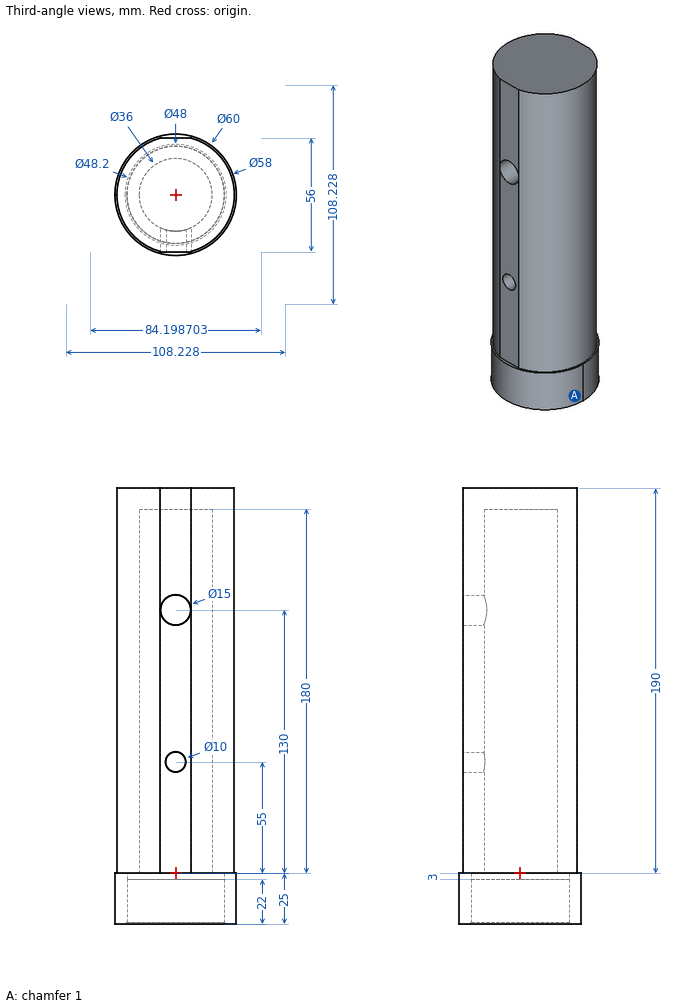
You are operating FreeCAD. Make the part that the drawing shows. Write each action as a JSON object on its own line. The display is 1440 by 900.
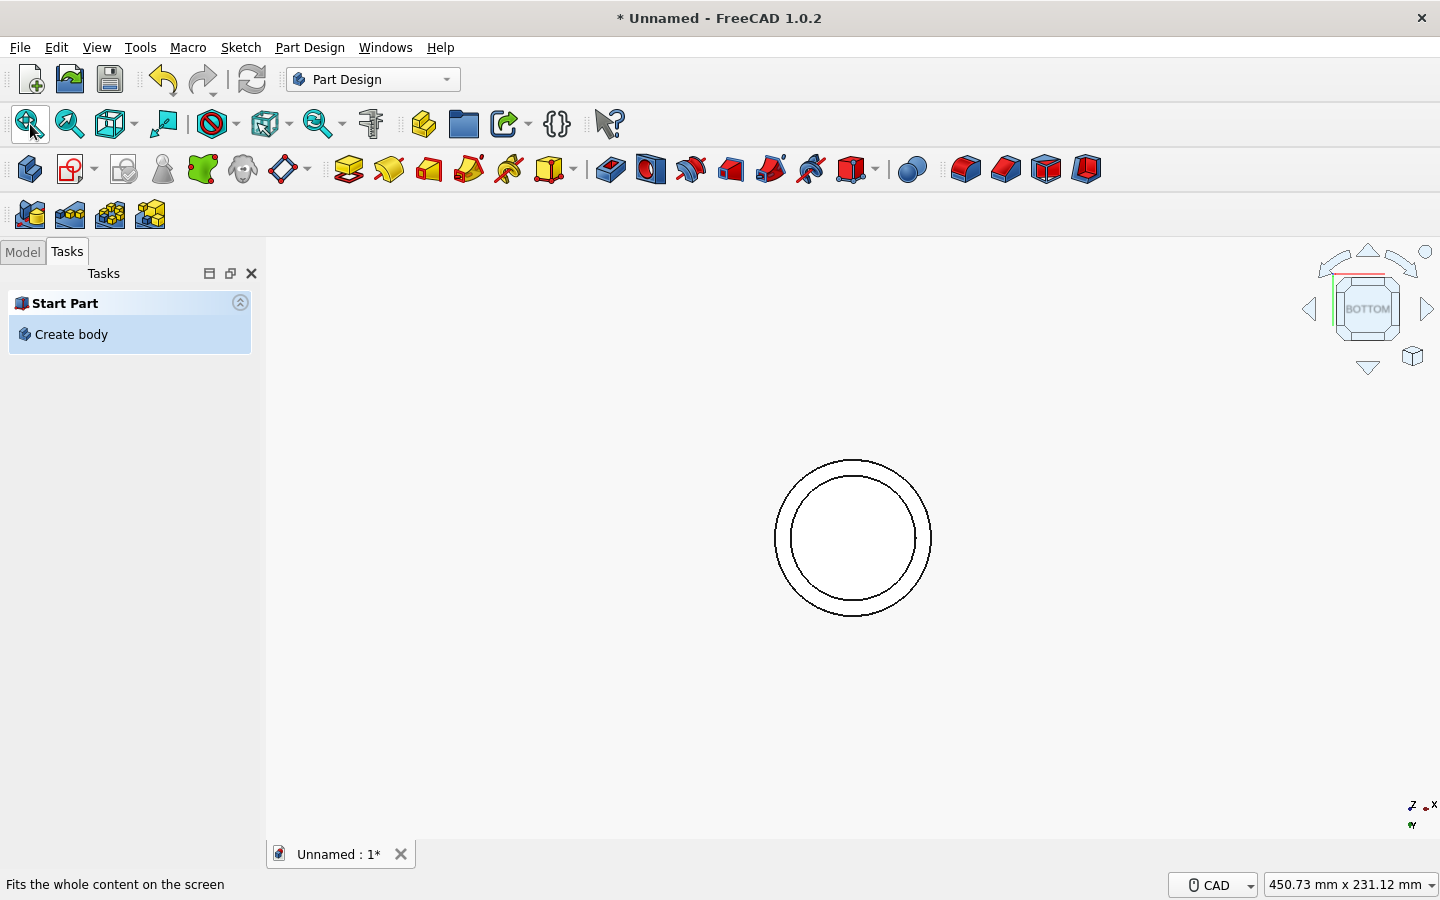
{"action": "left_click", "coordinate": [853, 537]}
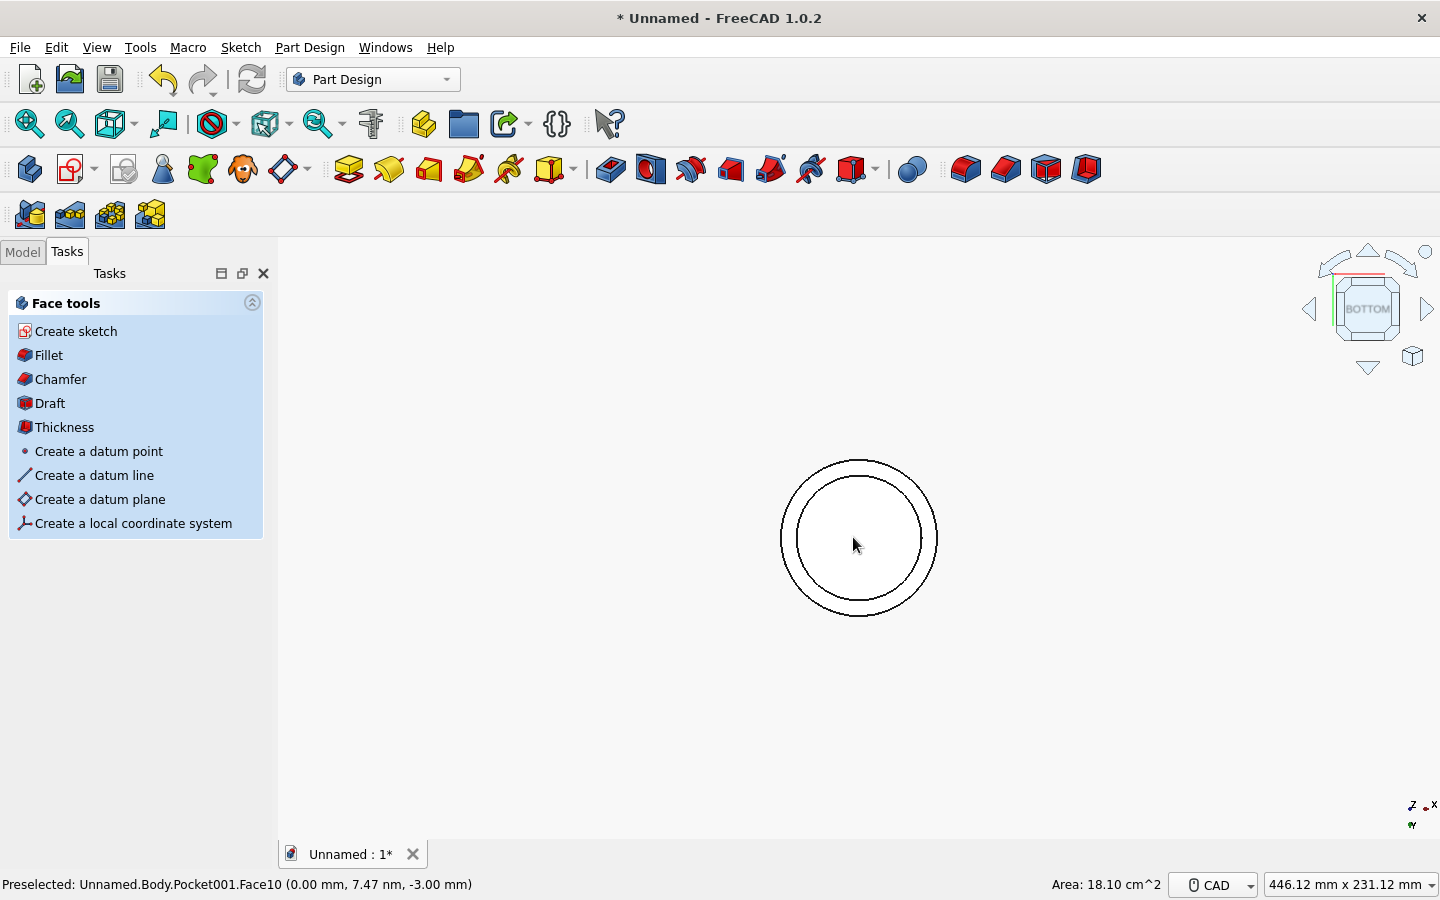
{"action": "left_click", "coordinate": [70, 170]}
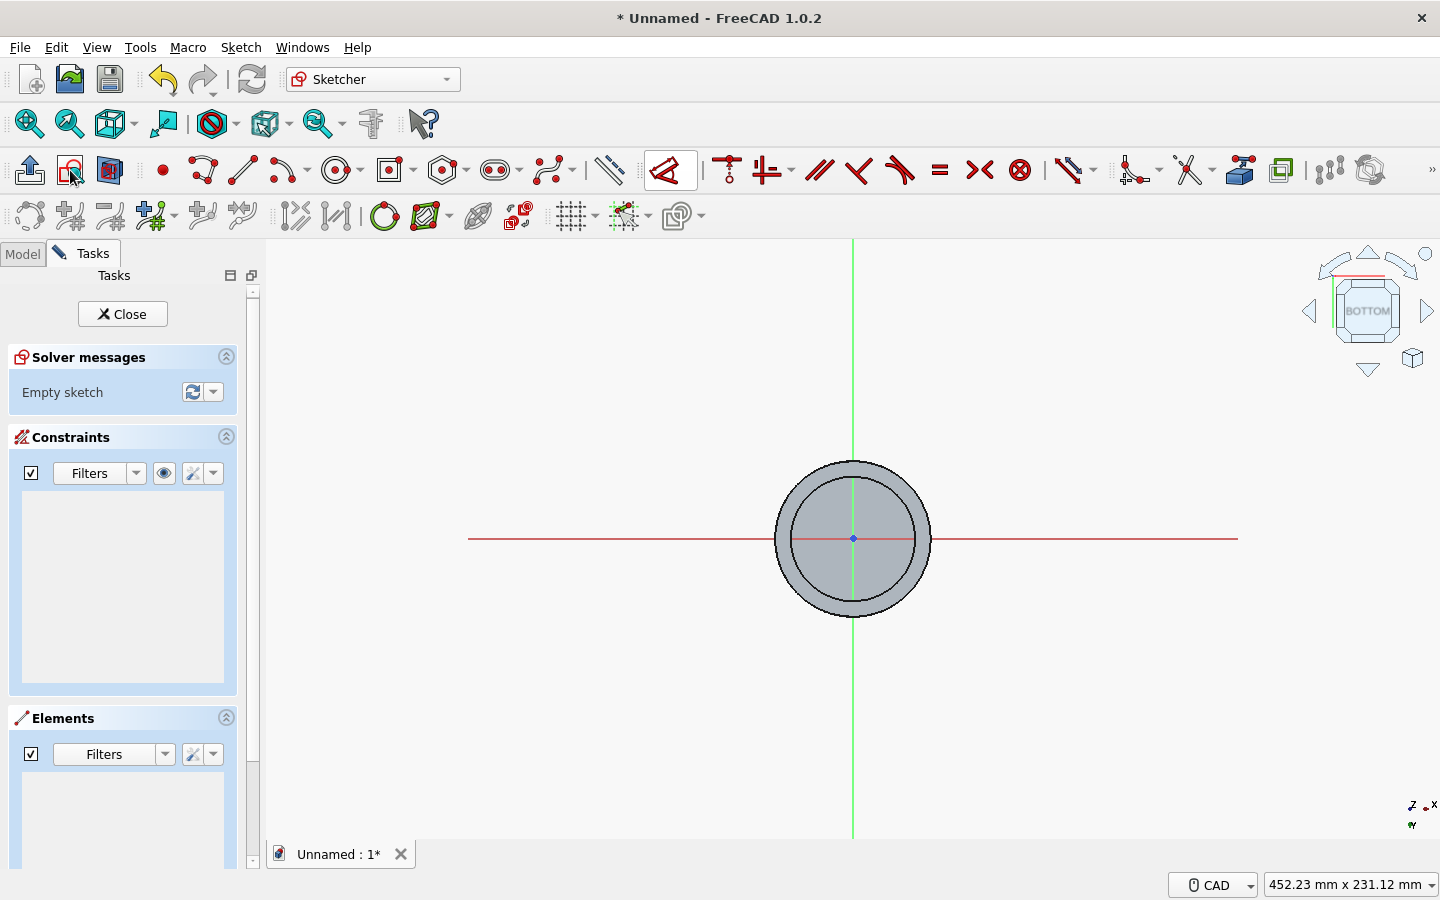
{"action": "scroll", "coordinate": [883, 539], "scroll_direction": "up", "scroll_amount": 6}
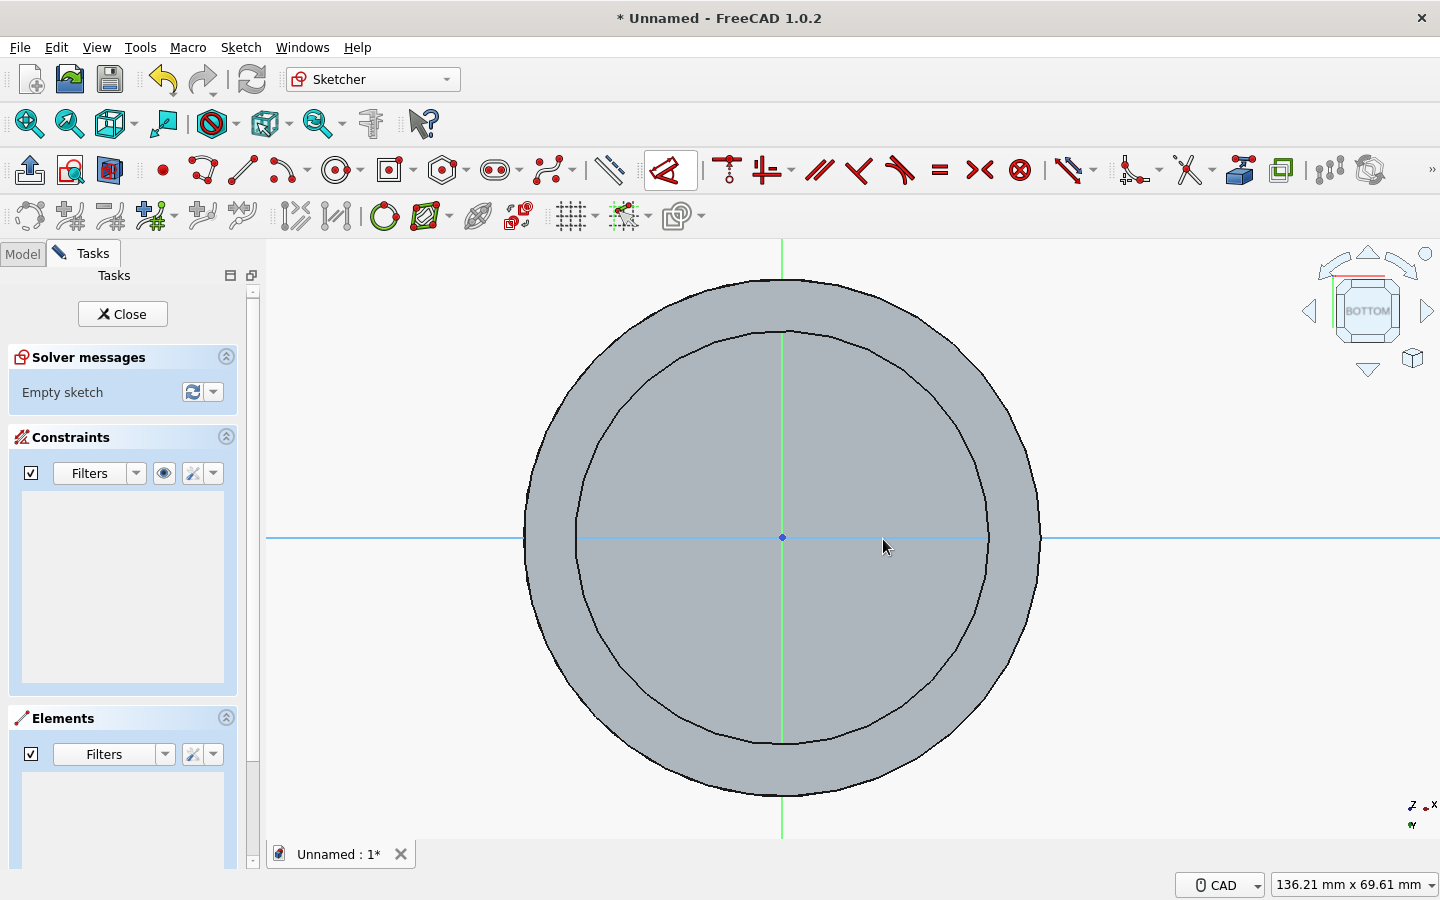
{"action": "left_click", "coordinate": [336, 170]}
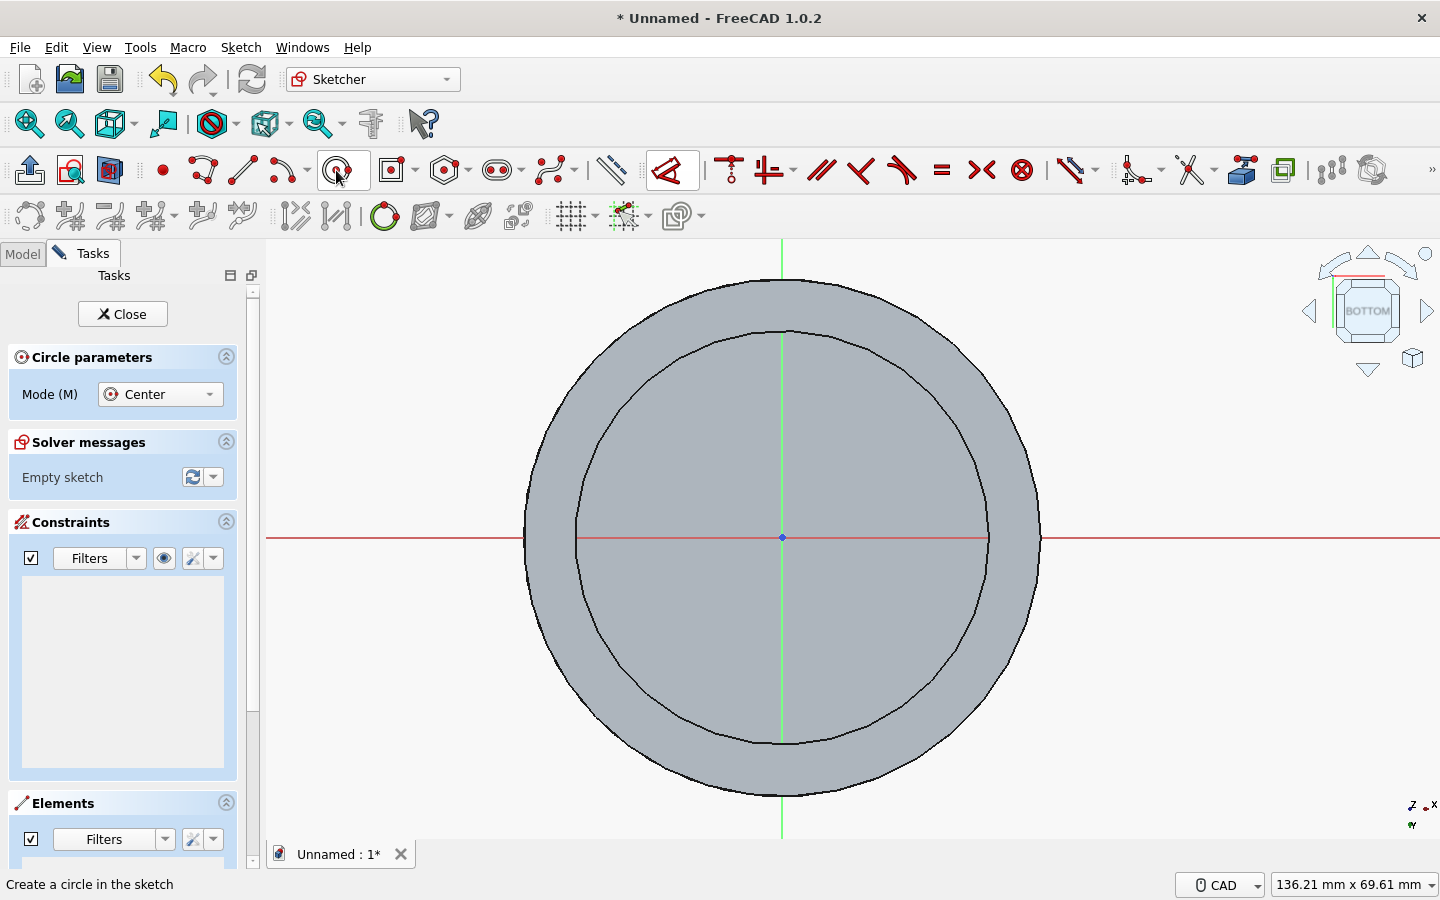
{"action": "left_click", "coordinate": [782, 538]}
{"action": "left_click", "coordinate": [929, 391]}
{"action": "key", "text": "Escape"}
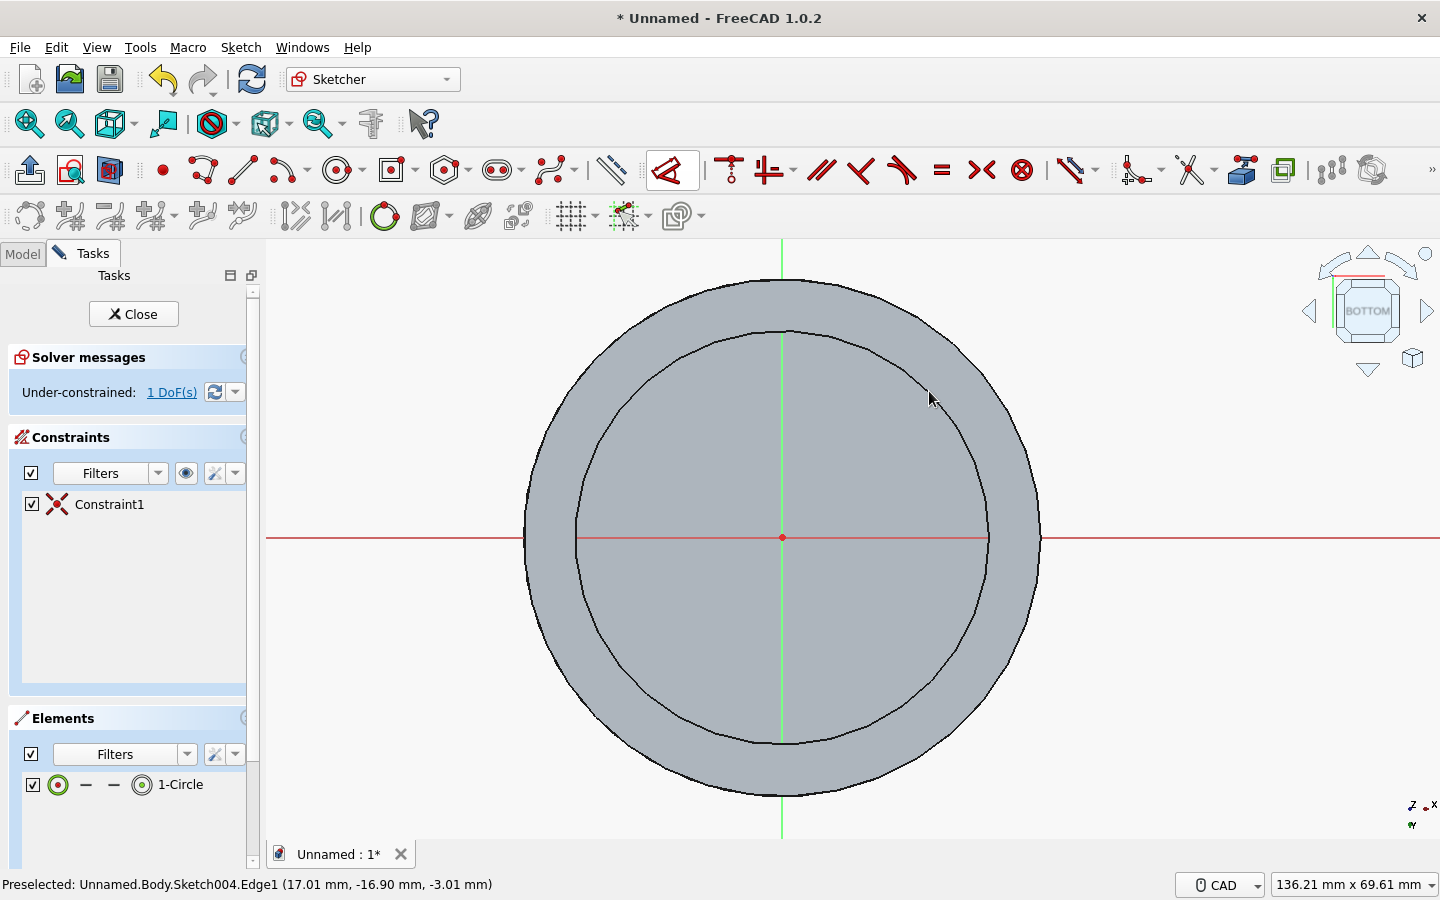
{"action": "left_click", "coordinate": [928, 391]}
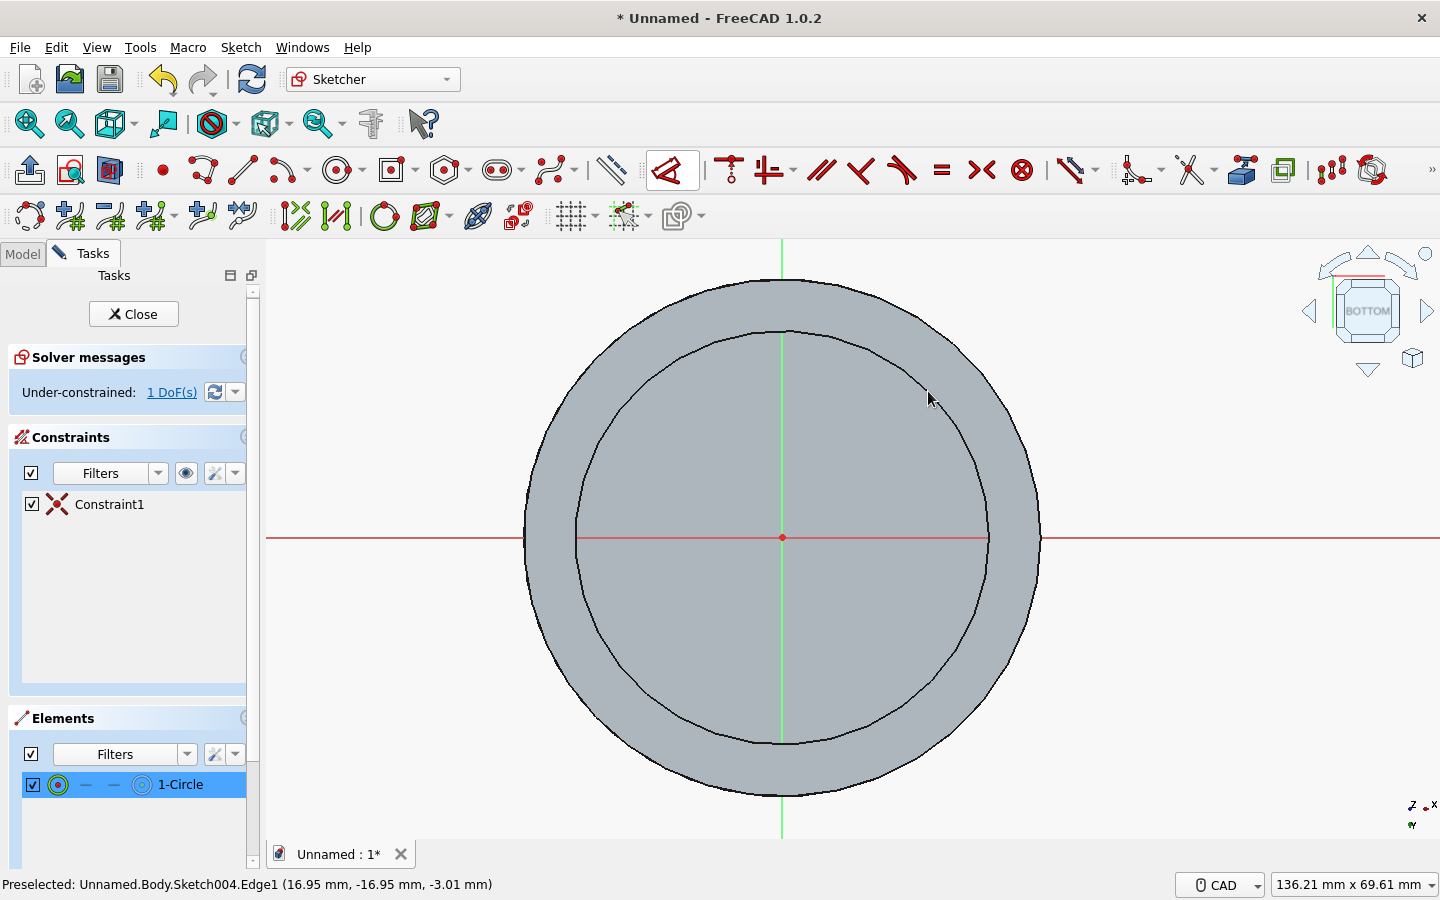
{"action": "key", "text": "k o"}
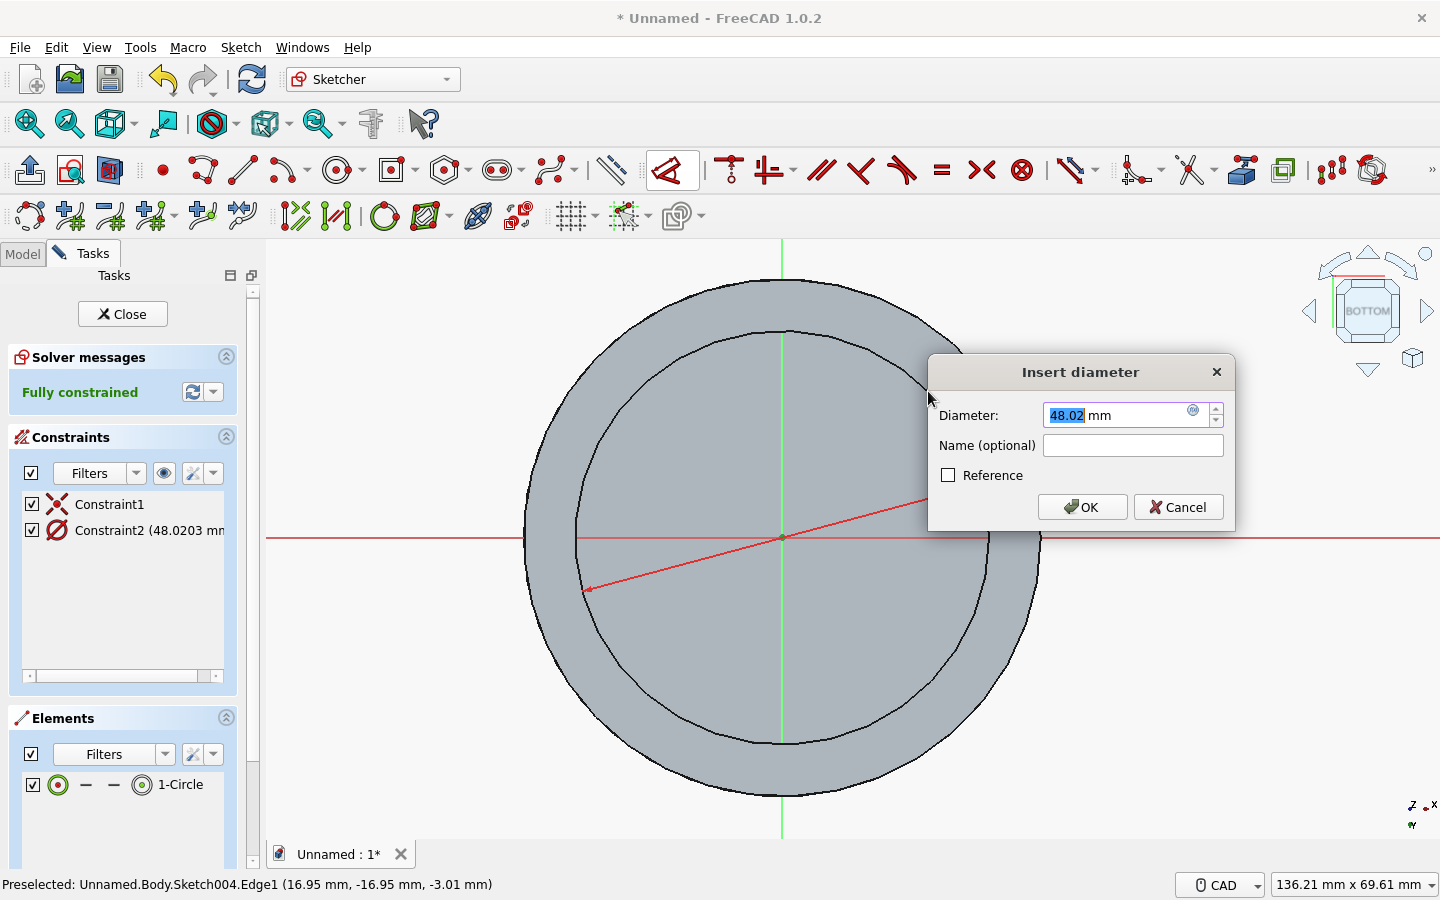
{"action": "type", "text": "48.2"}
{"action": "key", "text": "Return"}